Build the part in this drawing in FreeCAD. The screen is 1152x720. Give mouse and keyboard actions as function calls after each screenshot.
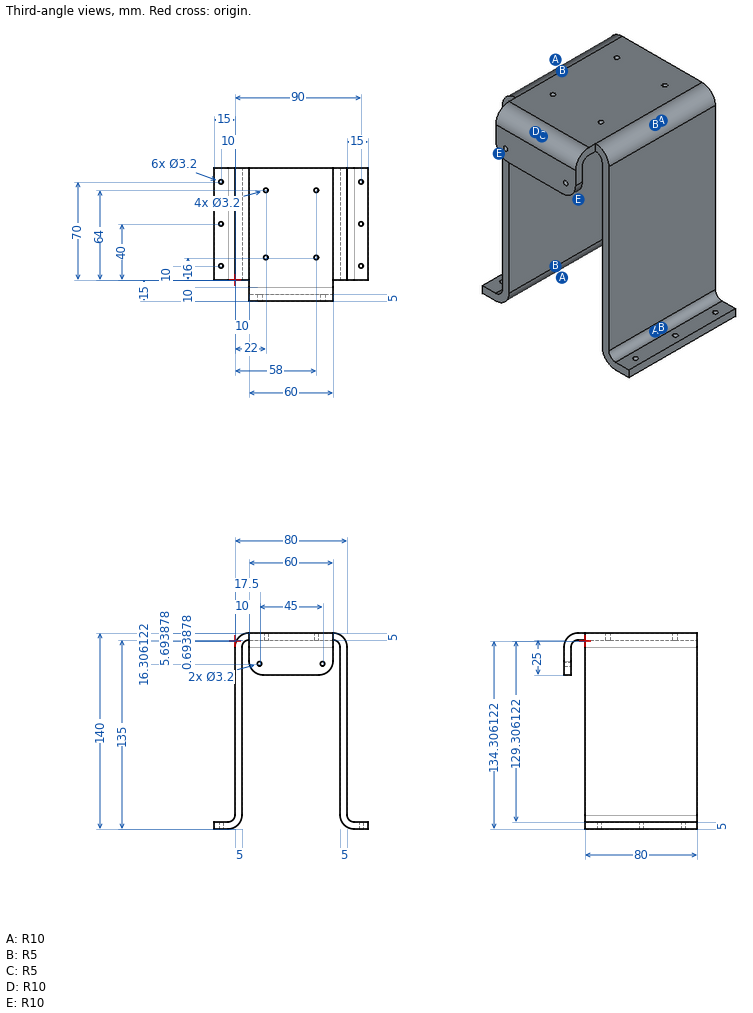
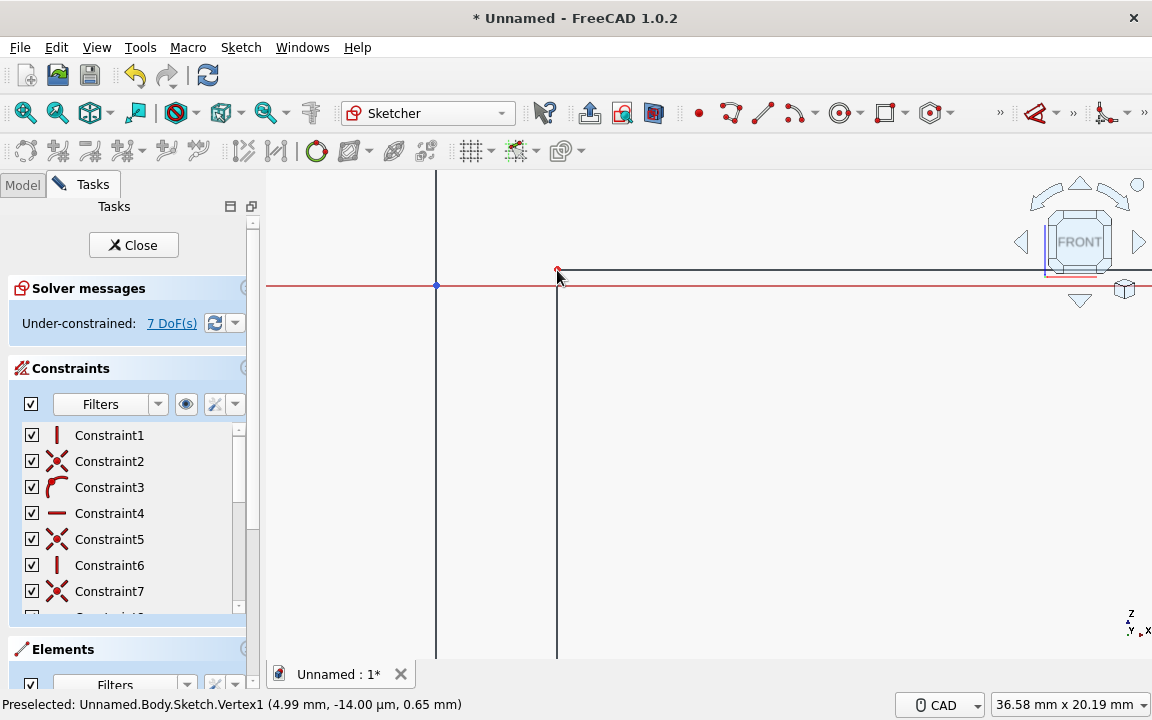
click(1036, 114)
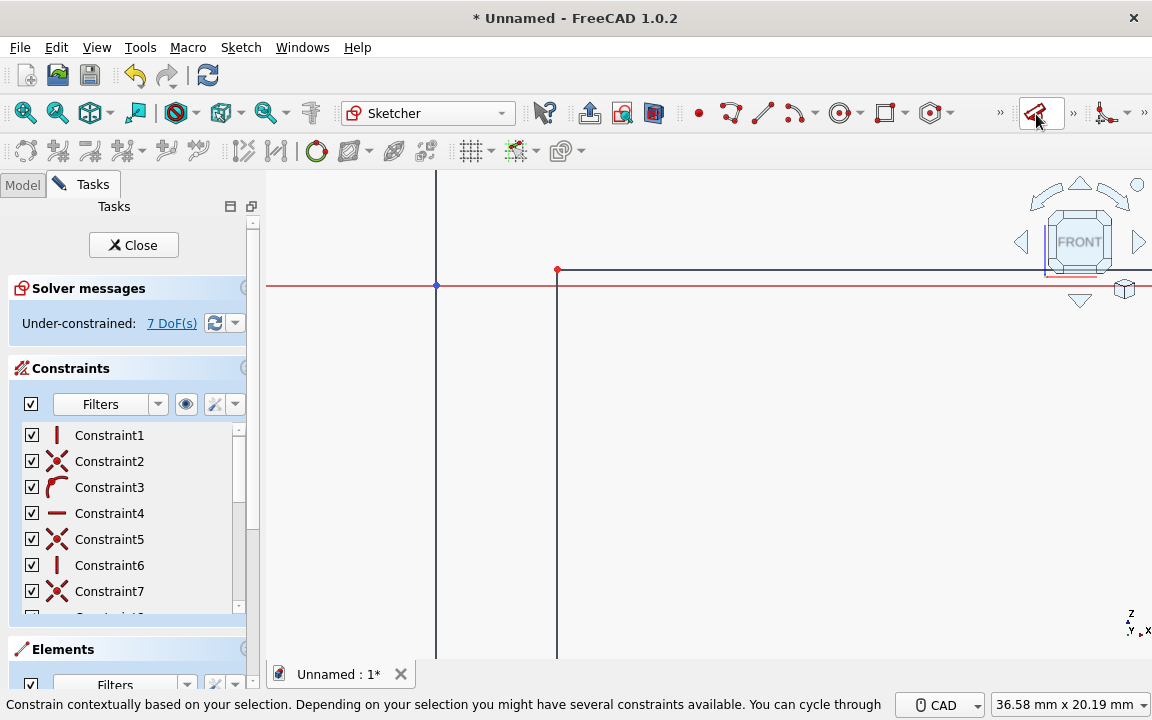
scroll(564, 272, down, 12)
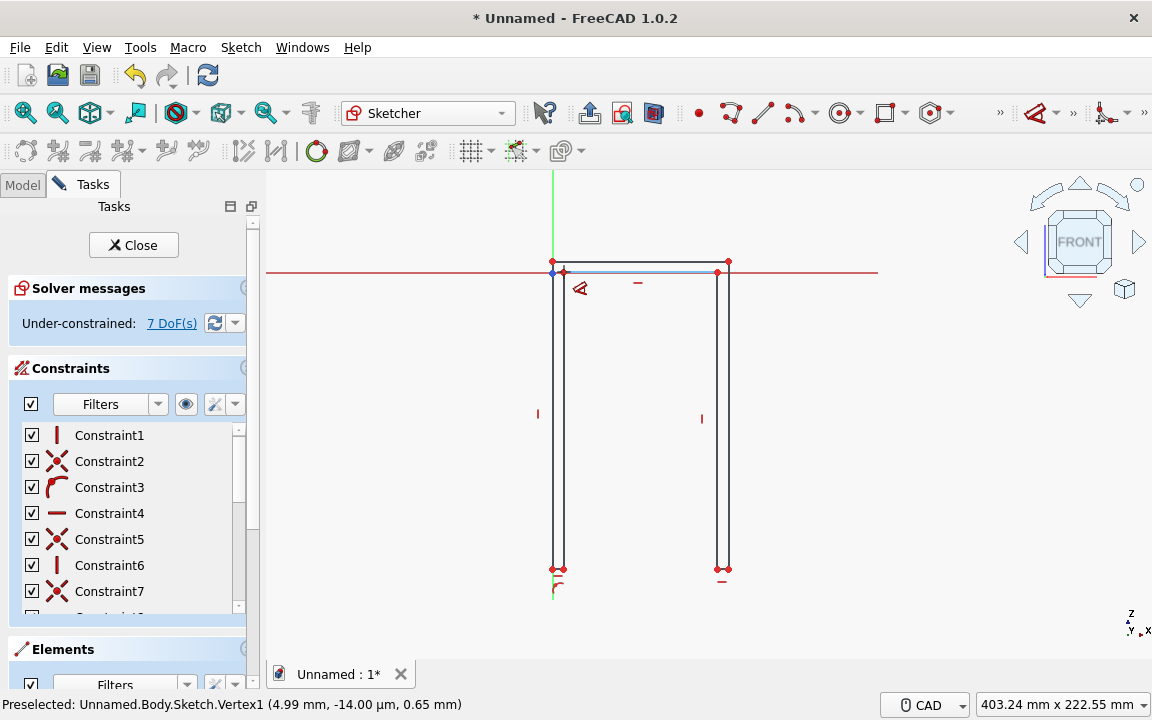
scroll(560, 569, up, 8)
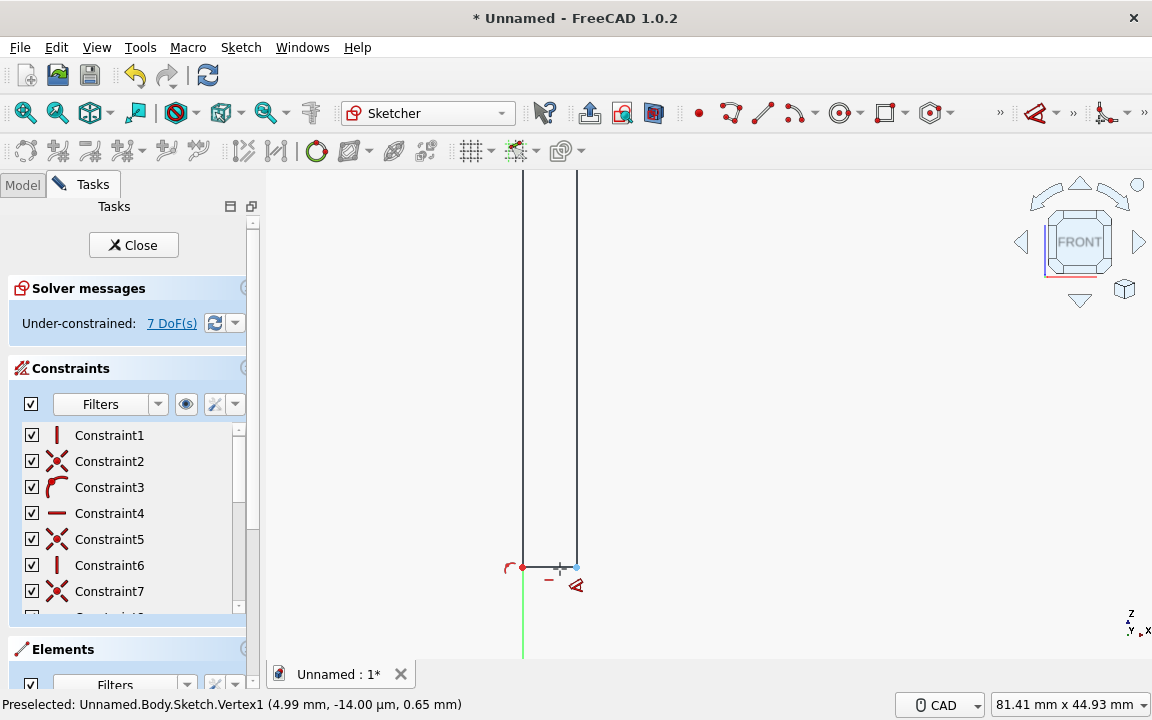
click(561, 567)
click(550, 601)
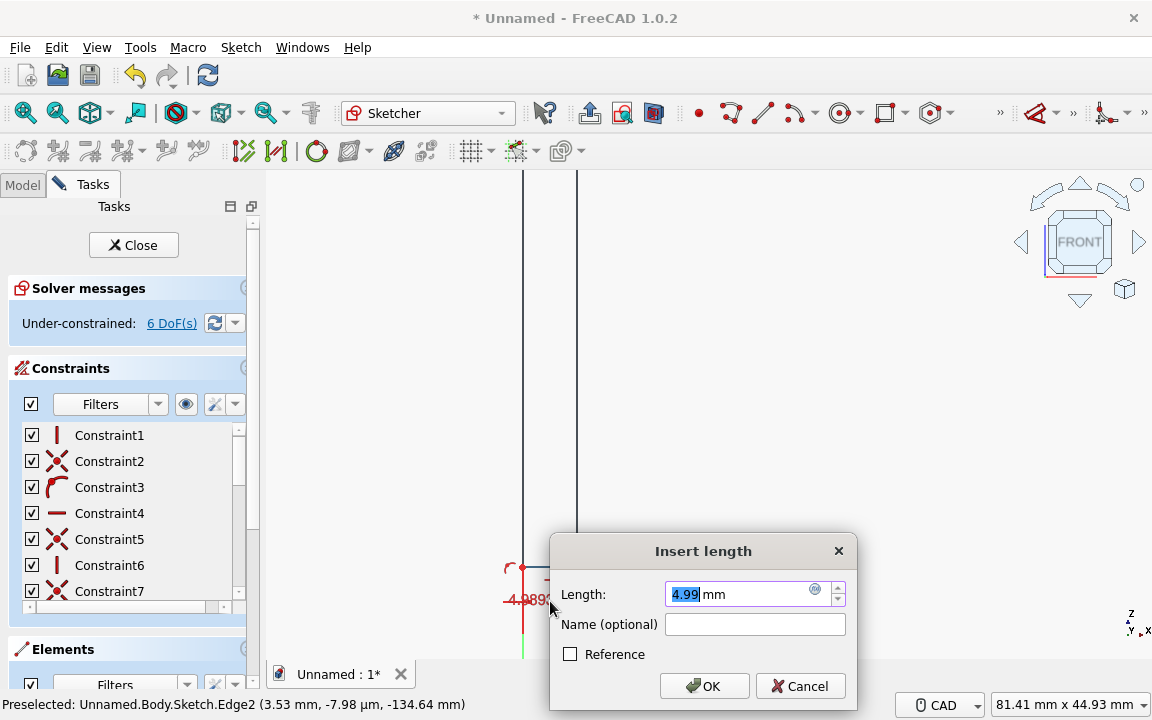
text(5)
key(Return)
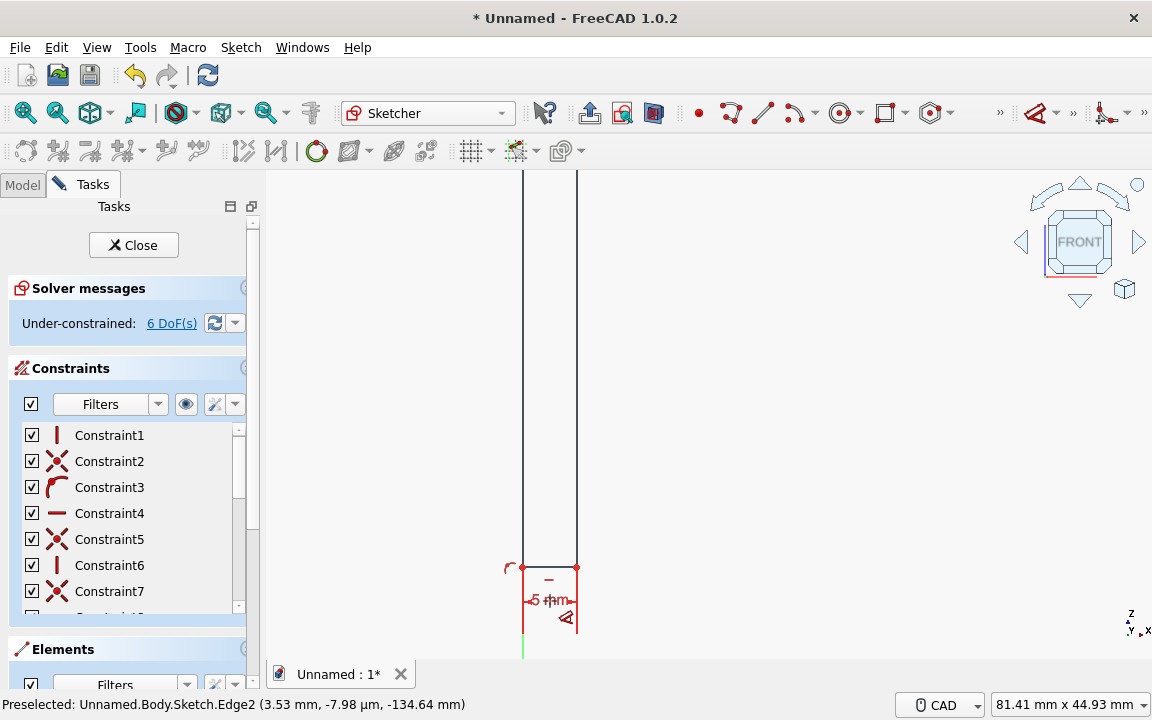
scroll(560, 570, down, 8)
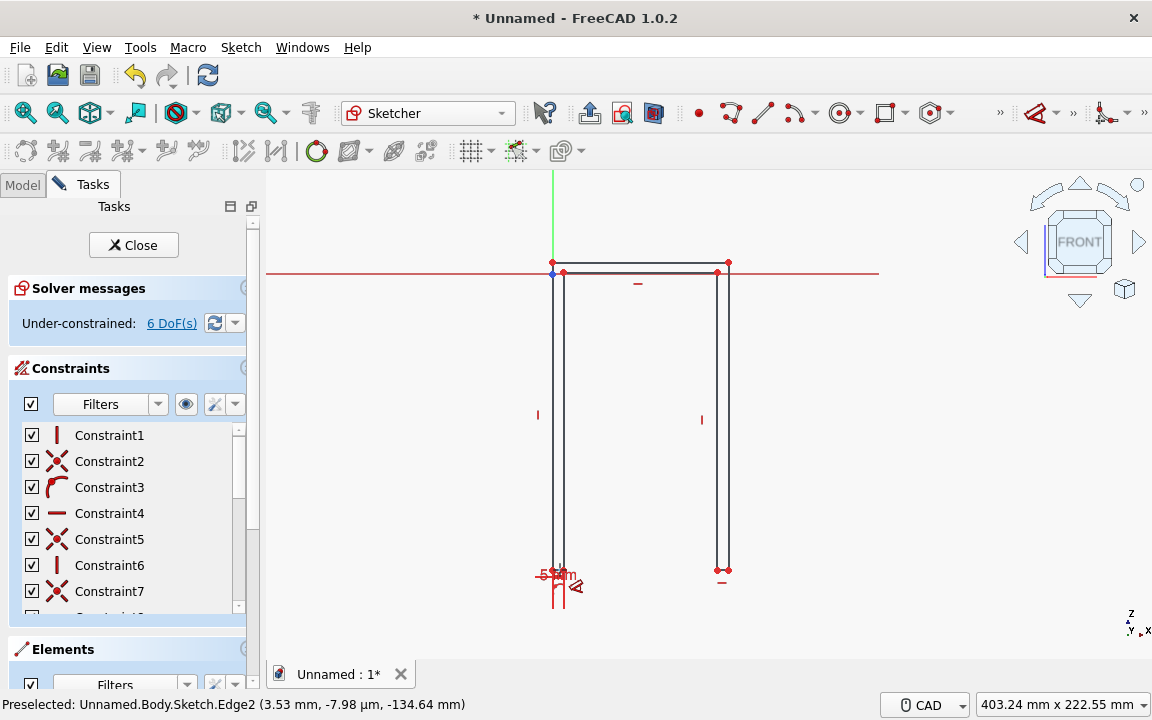
scroll(725, 570, up, 7)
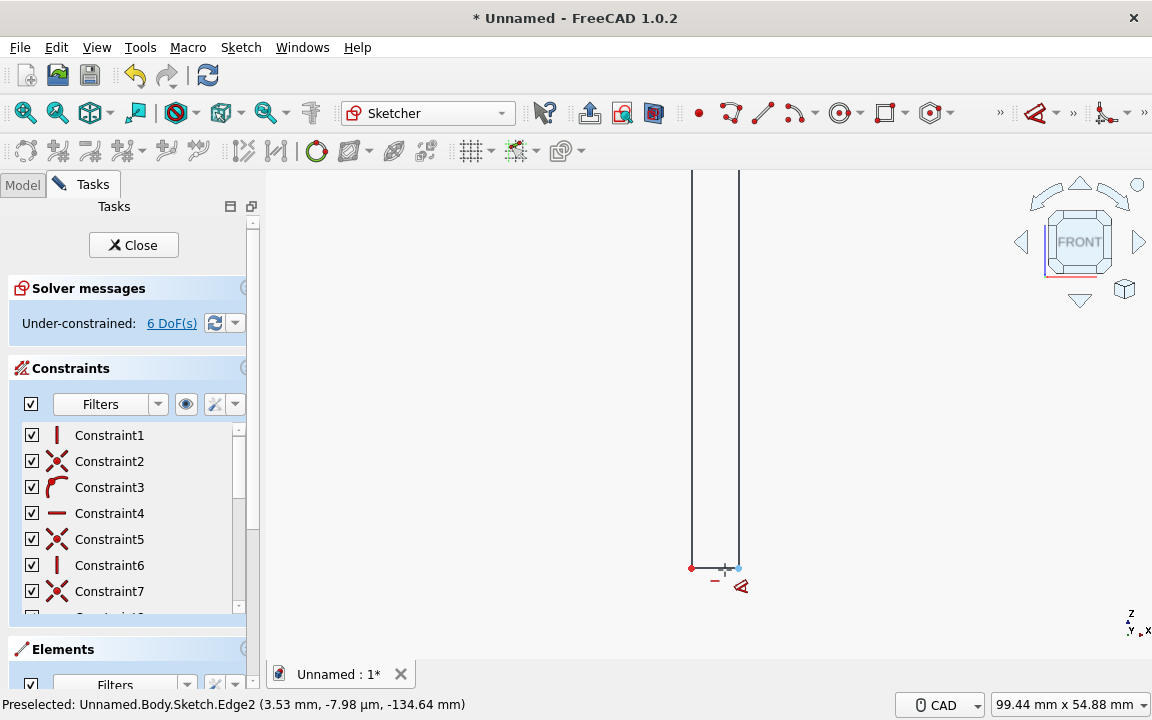
click(724, 568)
click(715, 602)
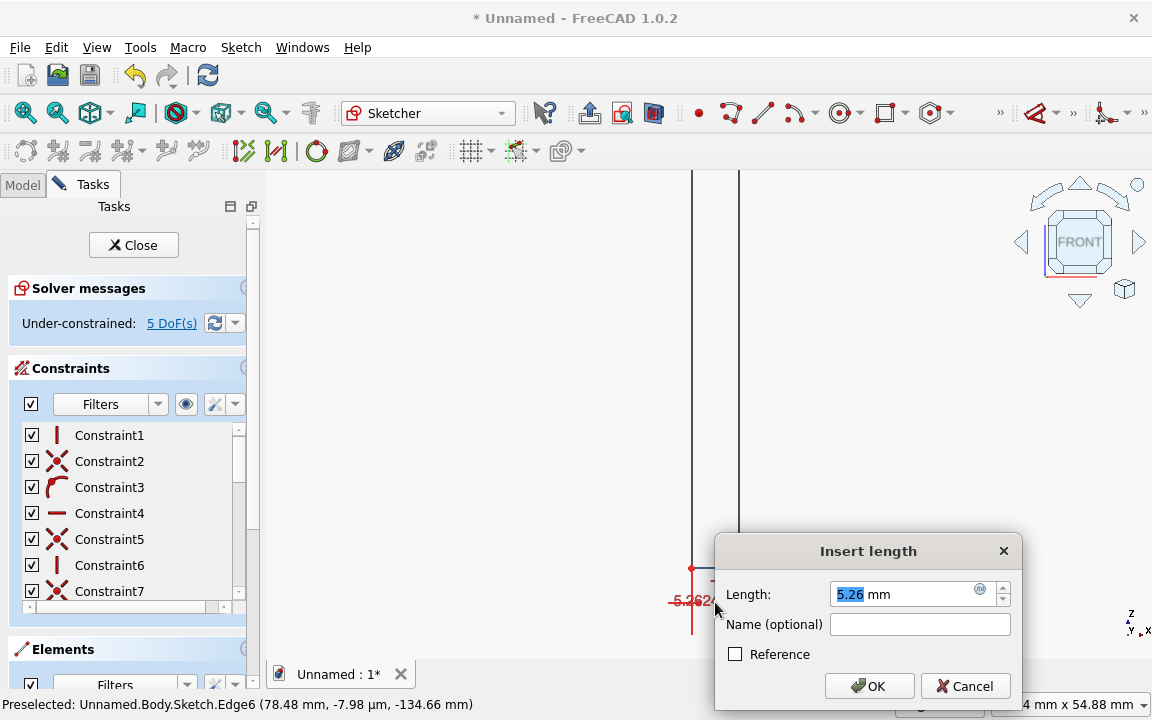
text(5)
key(Return)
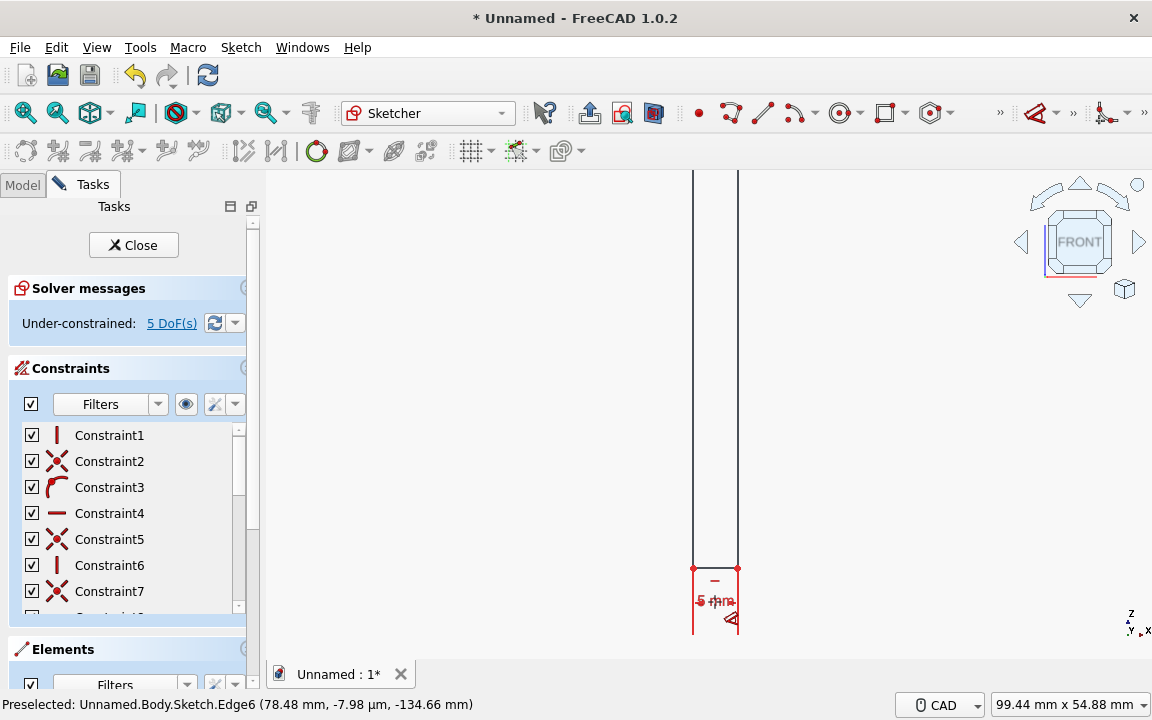
scroll(725, 569, down, 7)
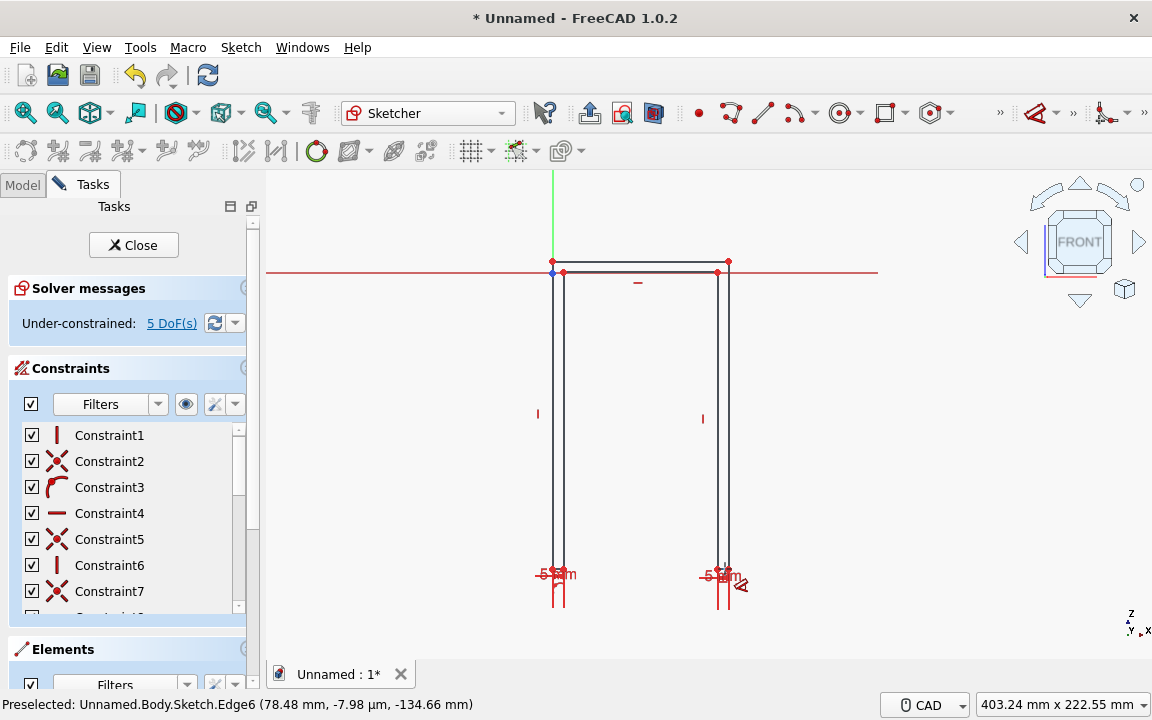
scroll(605, 262, up, 2)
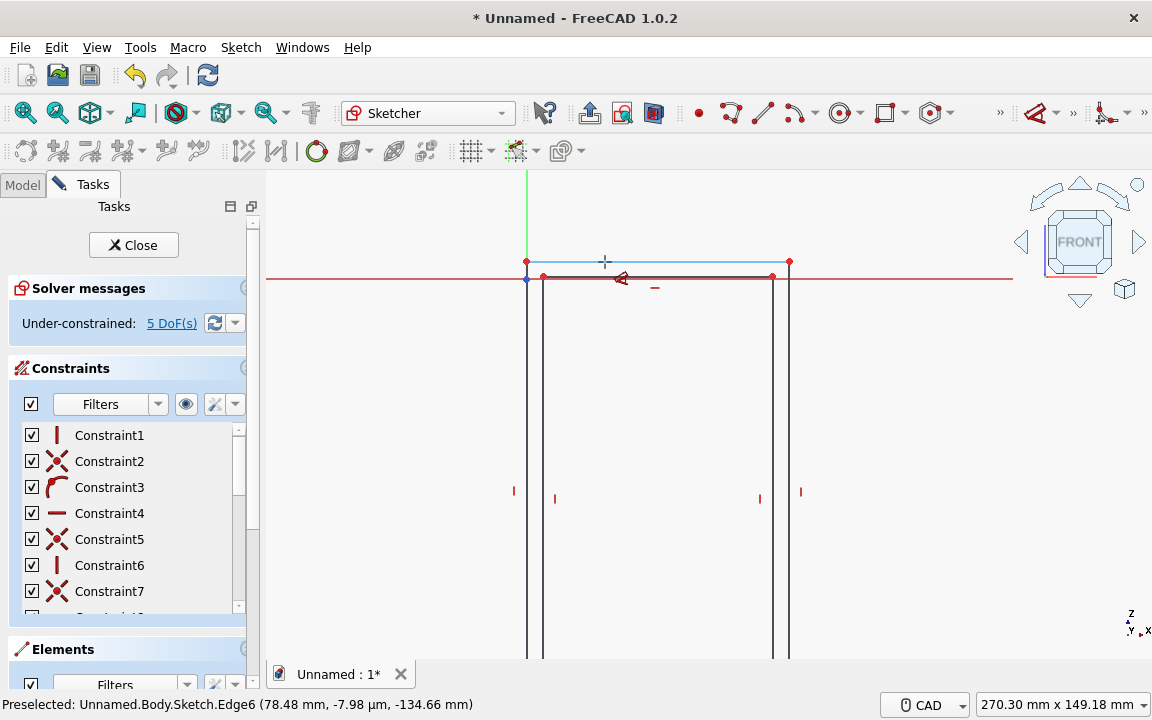
click(606, 262)
click(658, 228)